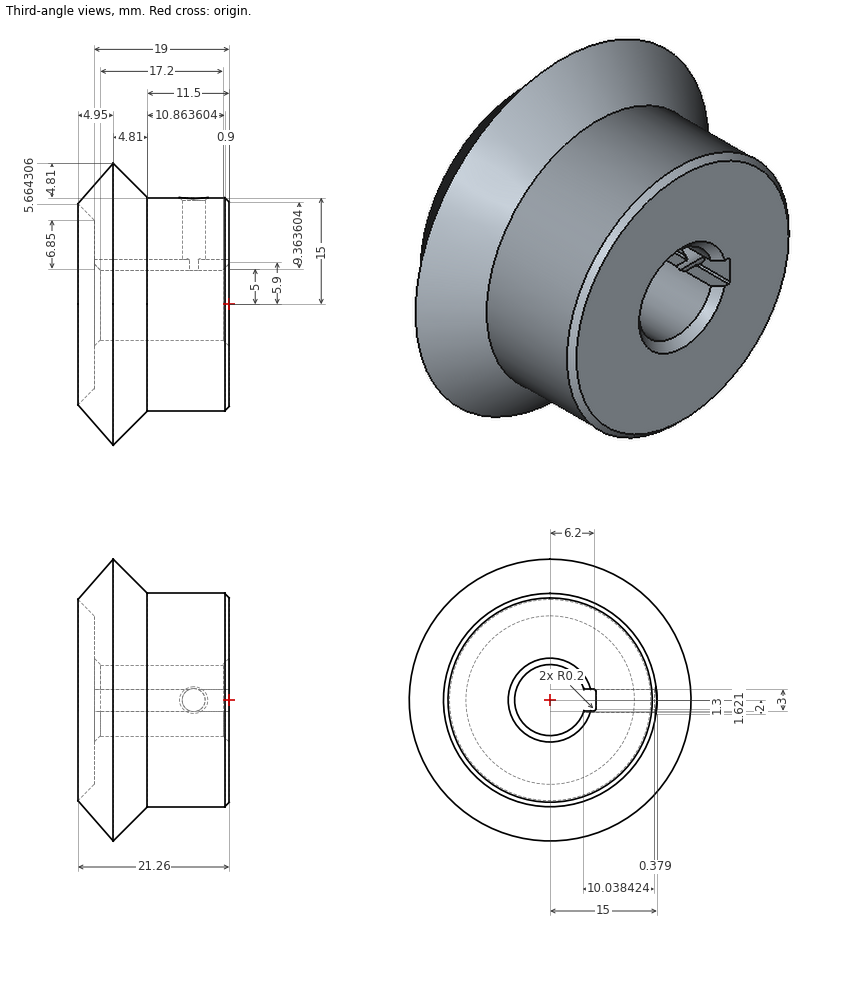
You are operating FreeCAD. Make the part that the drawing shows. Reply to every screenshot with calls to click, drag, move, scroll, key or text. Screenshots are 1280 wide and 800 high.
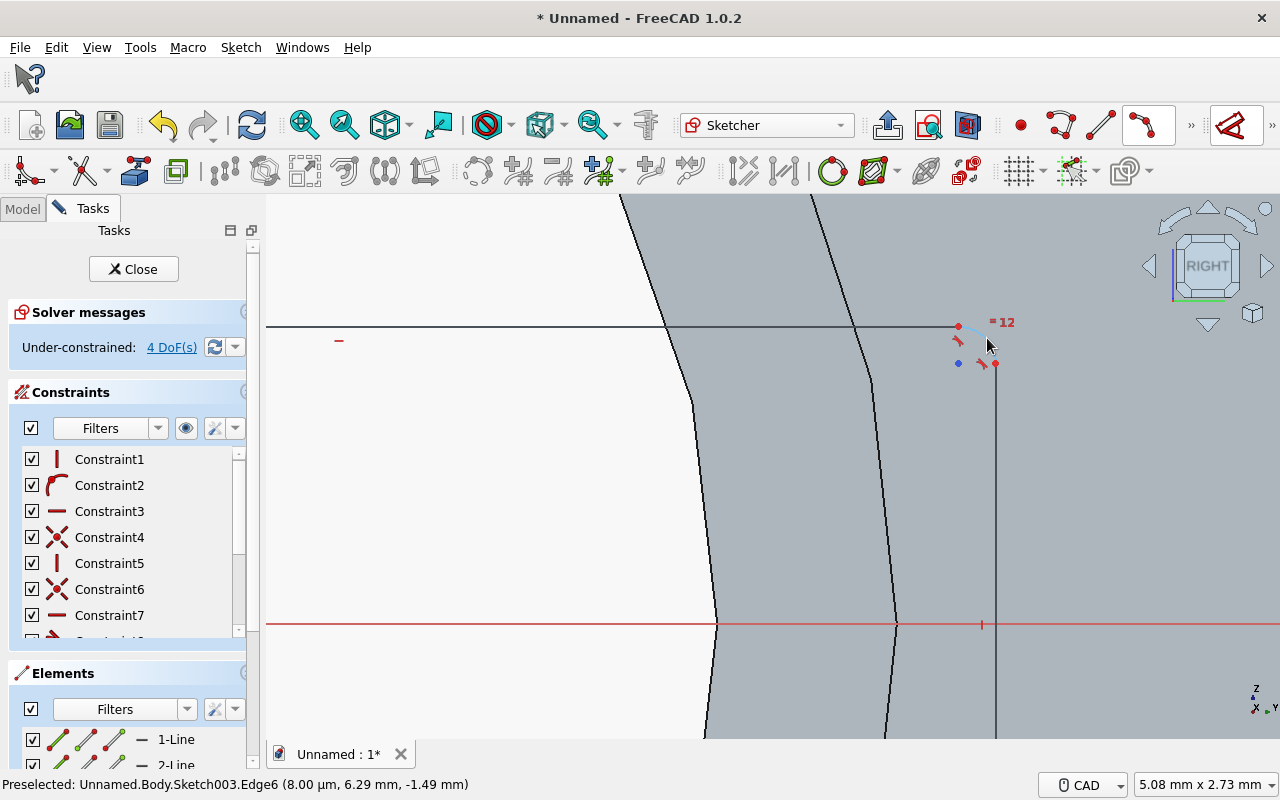
click(985, 338)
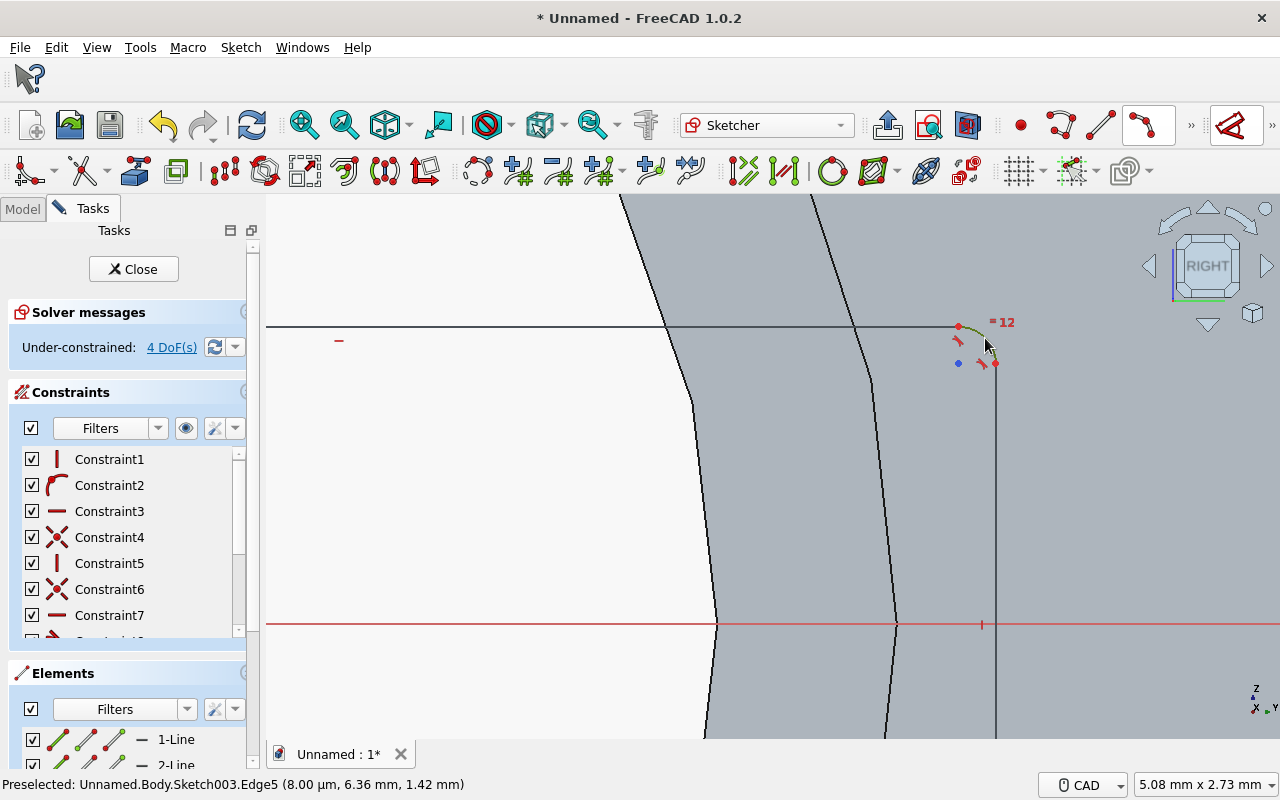
key(k)
key(r)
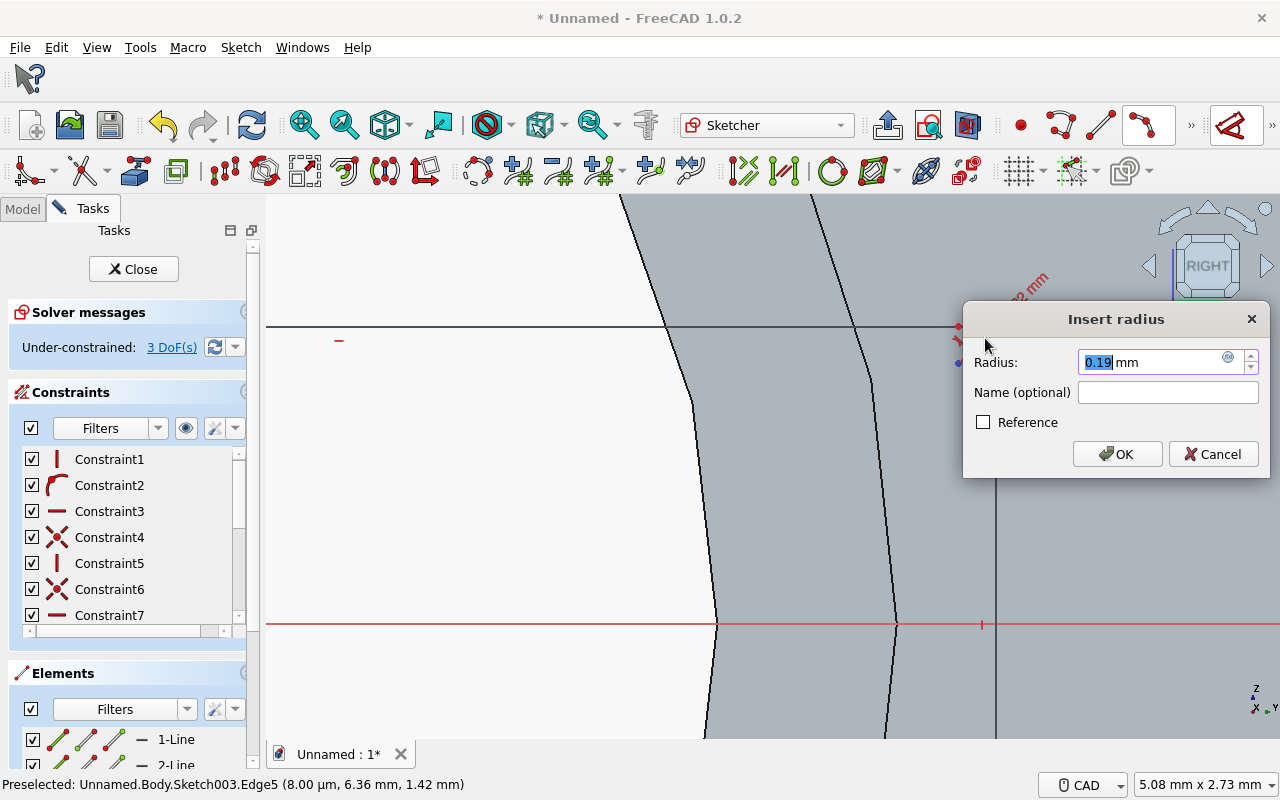
text(0.2)
key(Return)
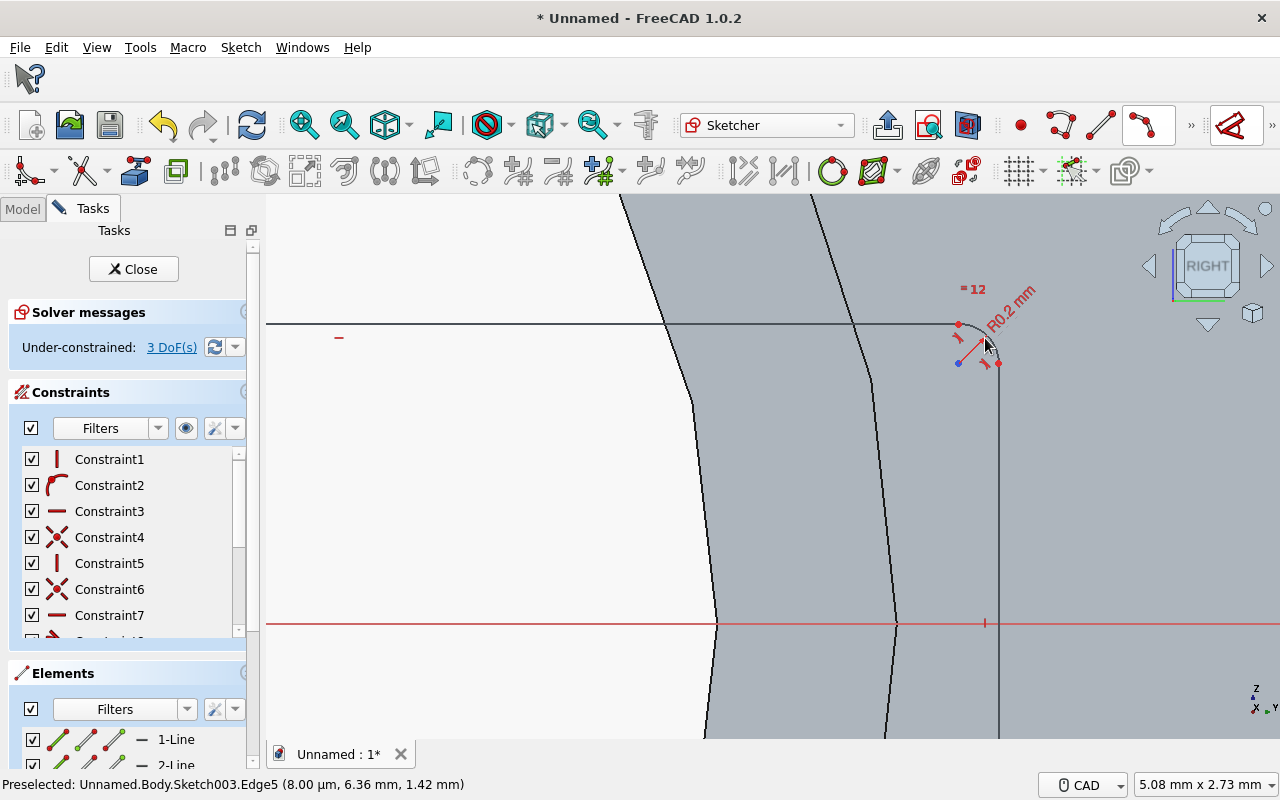
scroll(987, 338, down, 4)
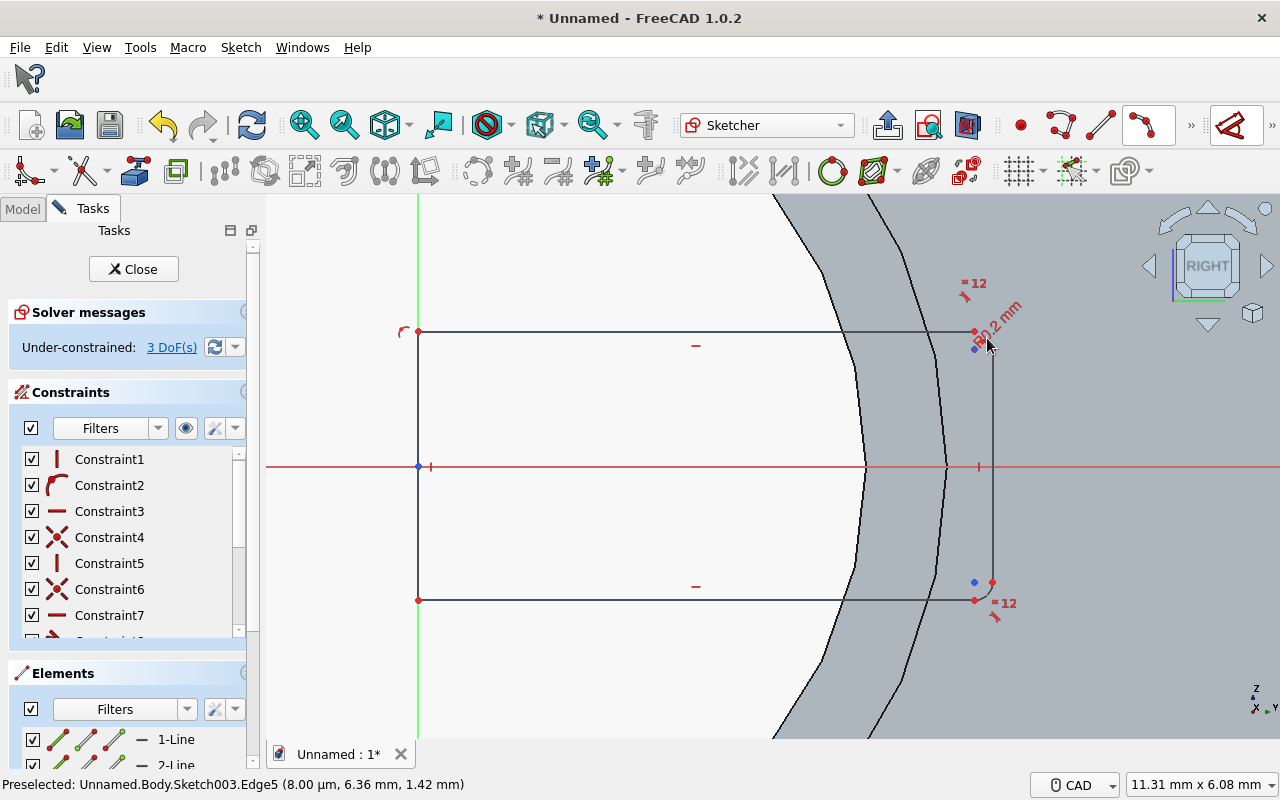
click(418, 412)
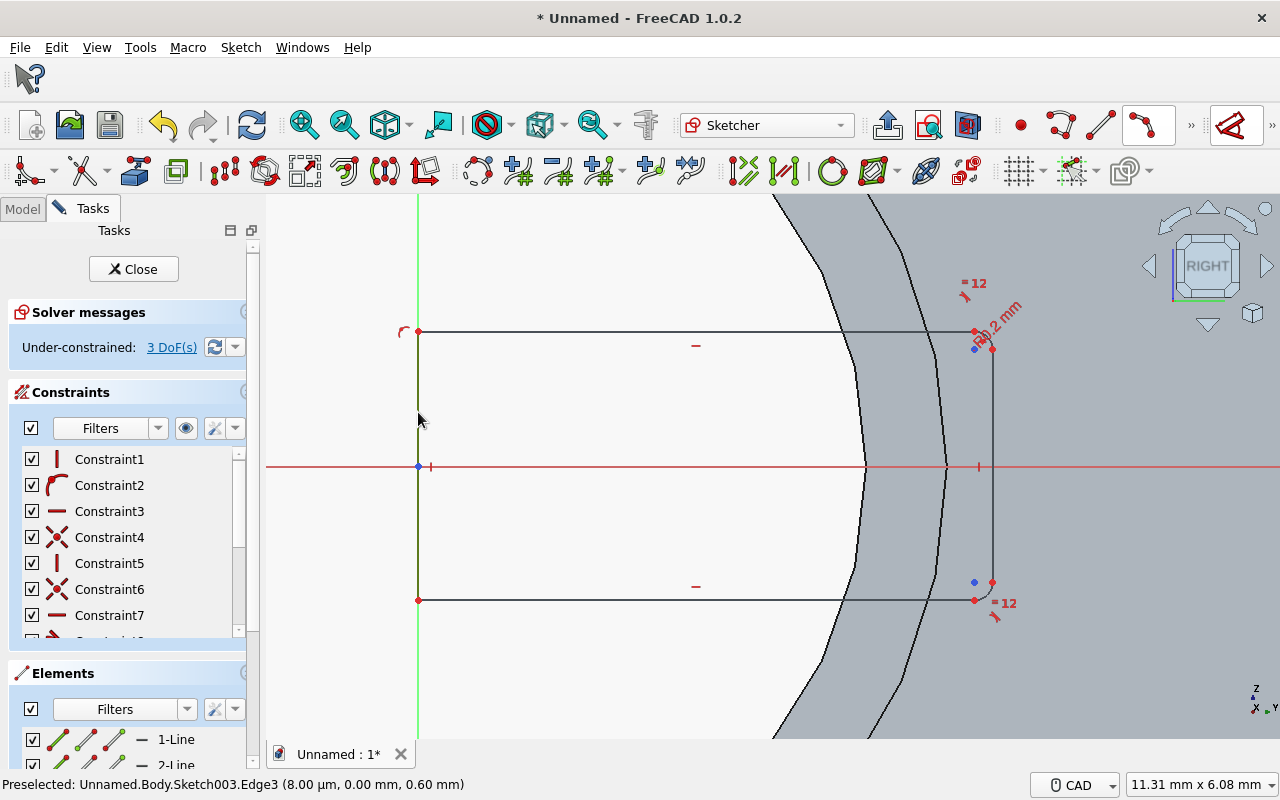
key(i)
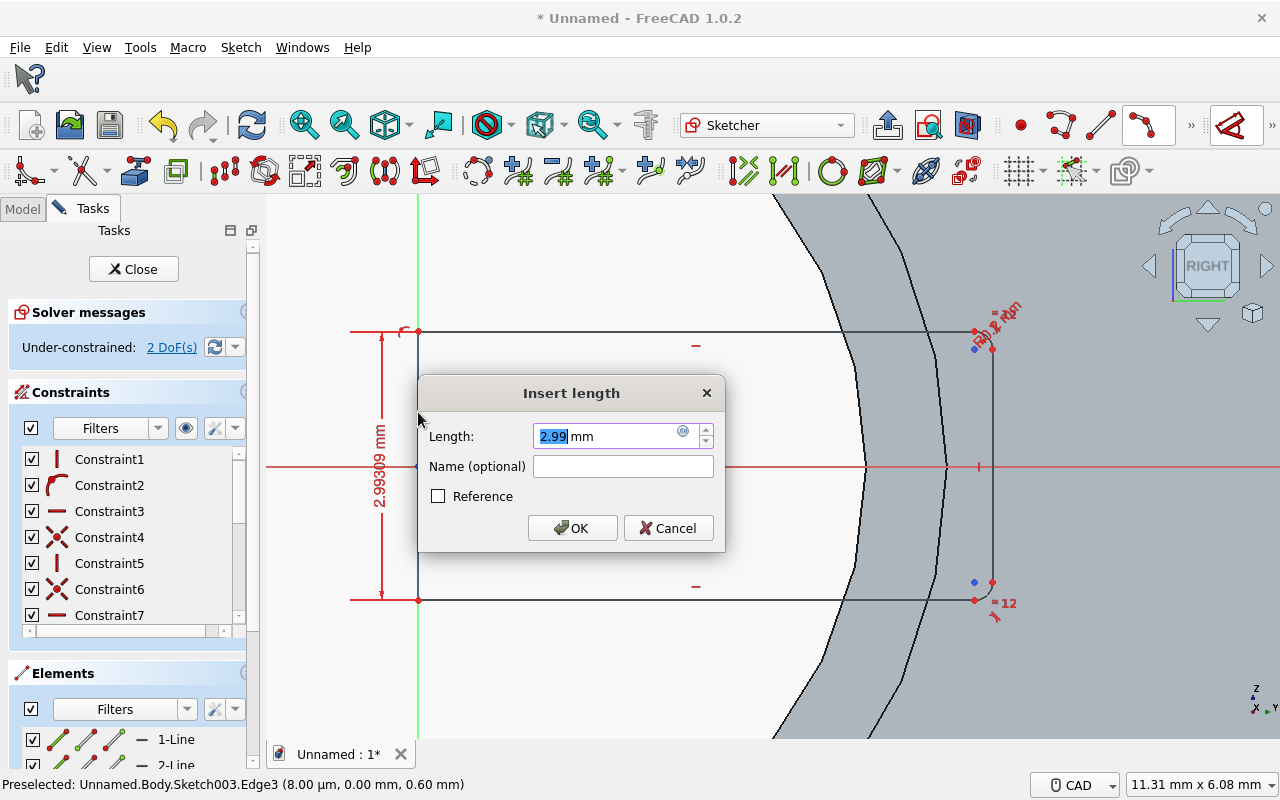
text(3)
key(Return)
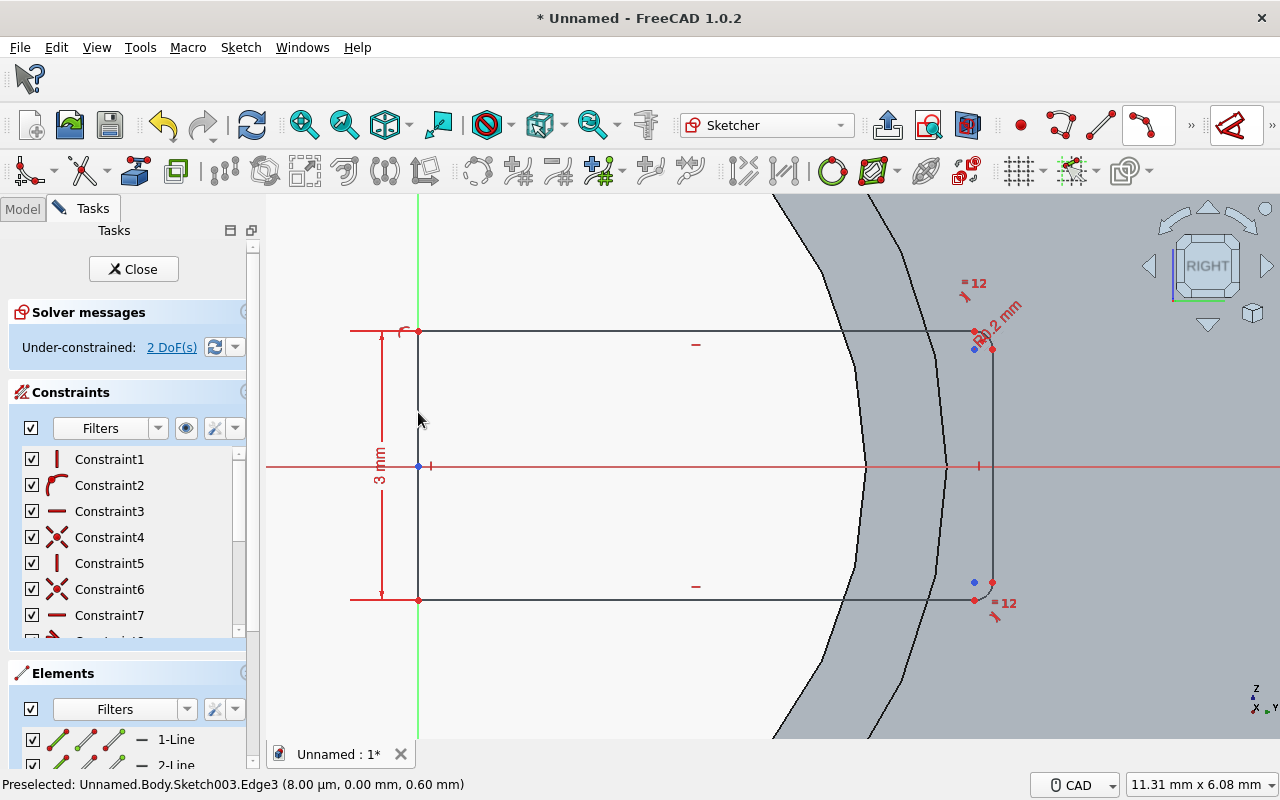
click(808, 331)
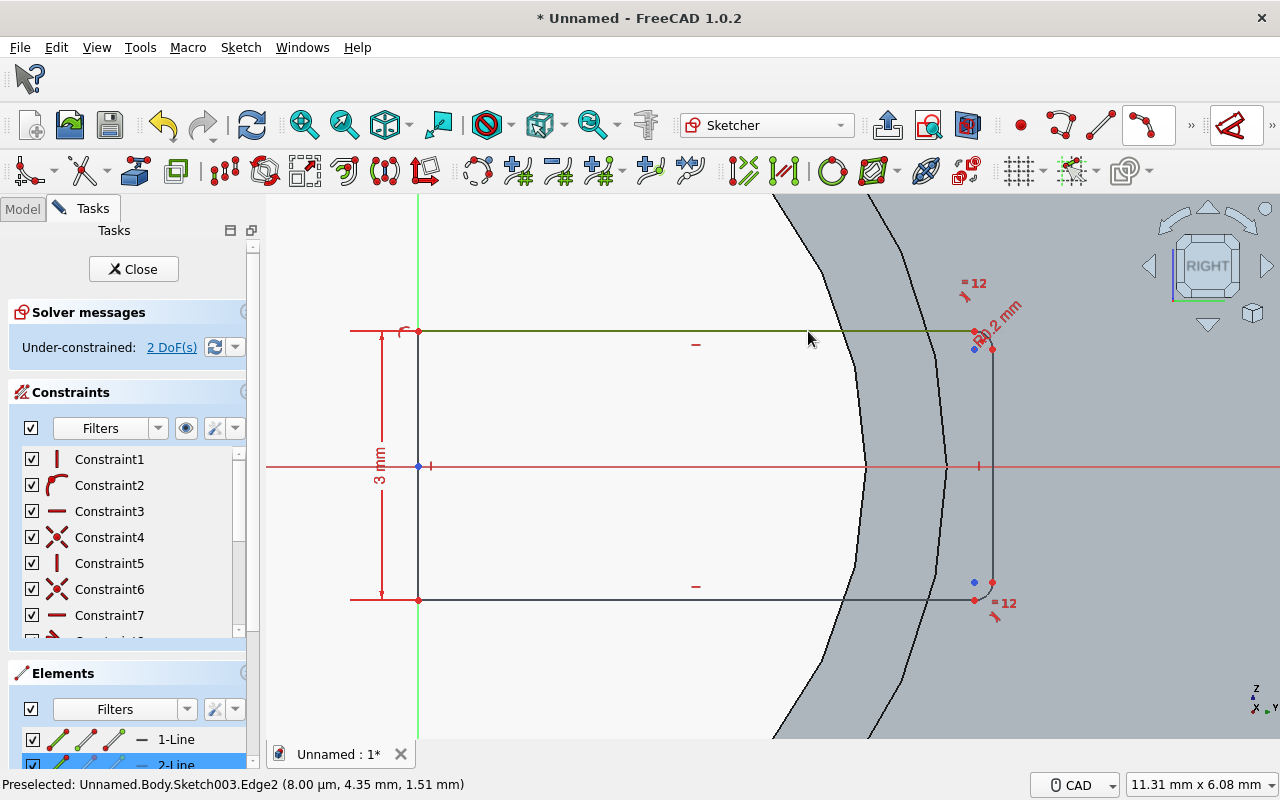
click(1258, 126)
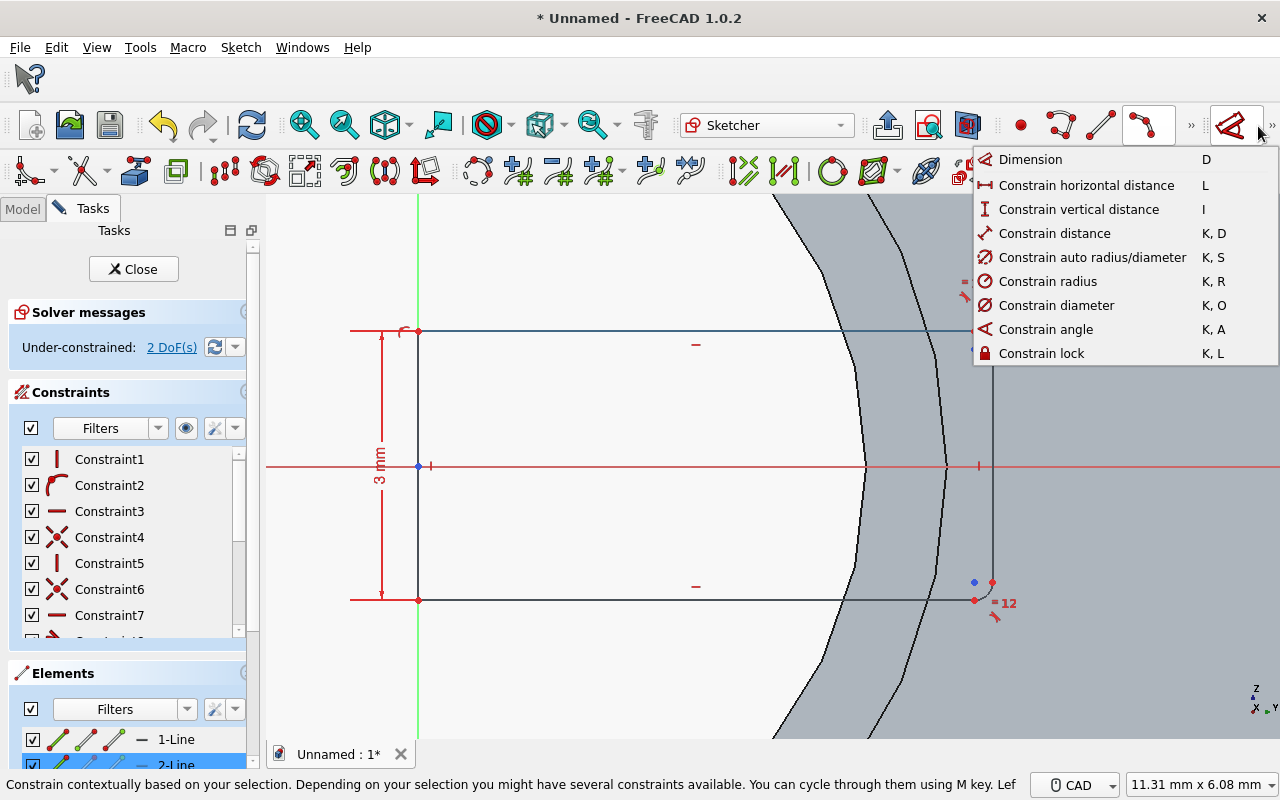
click(1126, 185)